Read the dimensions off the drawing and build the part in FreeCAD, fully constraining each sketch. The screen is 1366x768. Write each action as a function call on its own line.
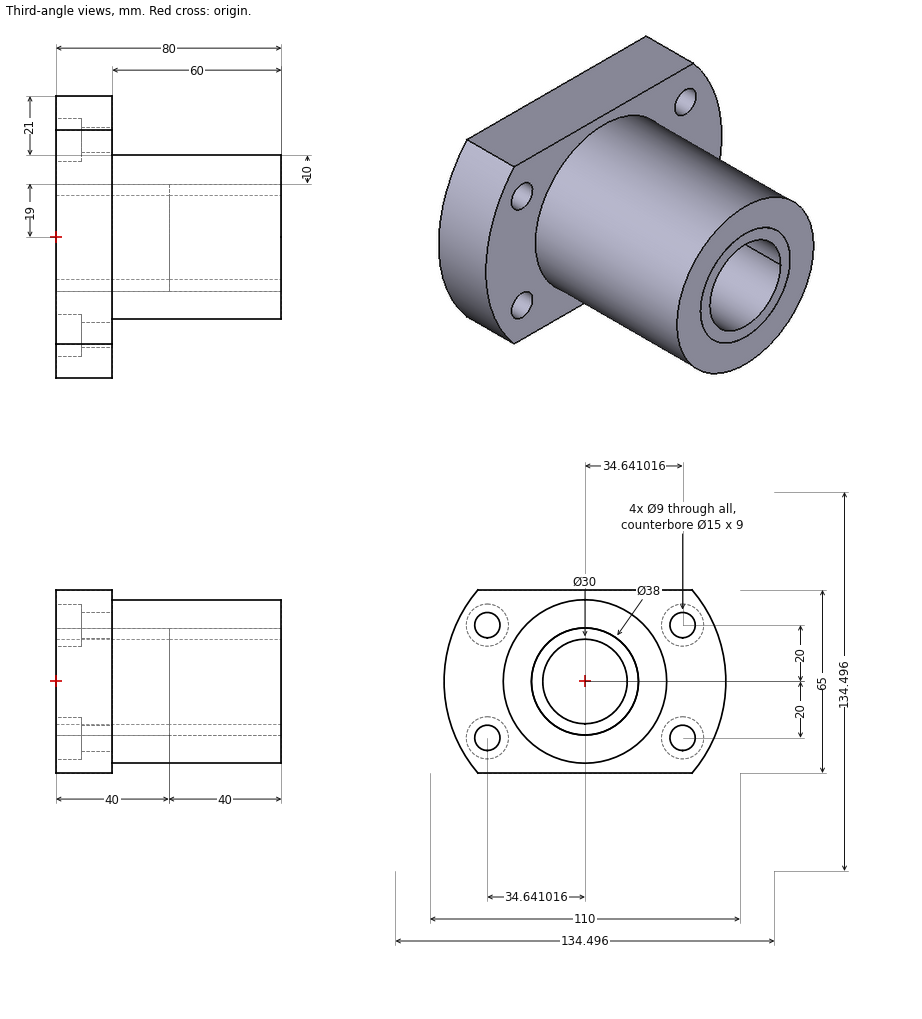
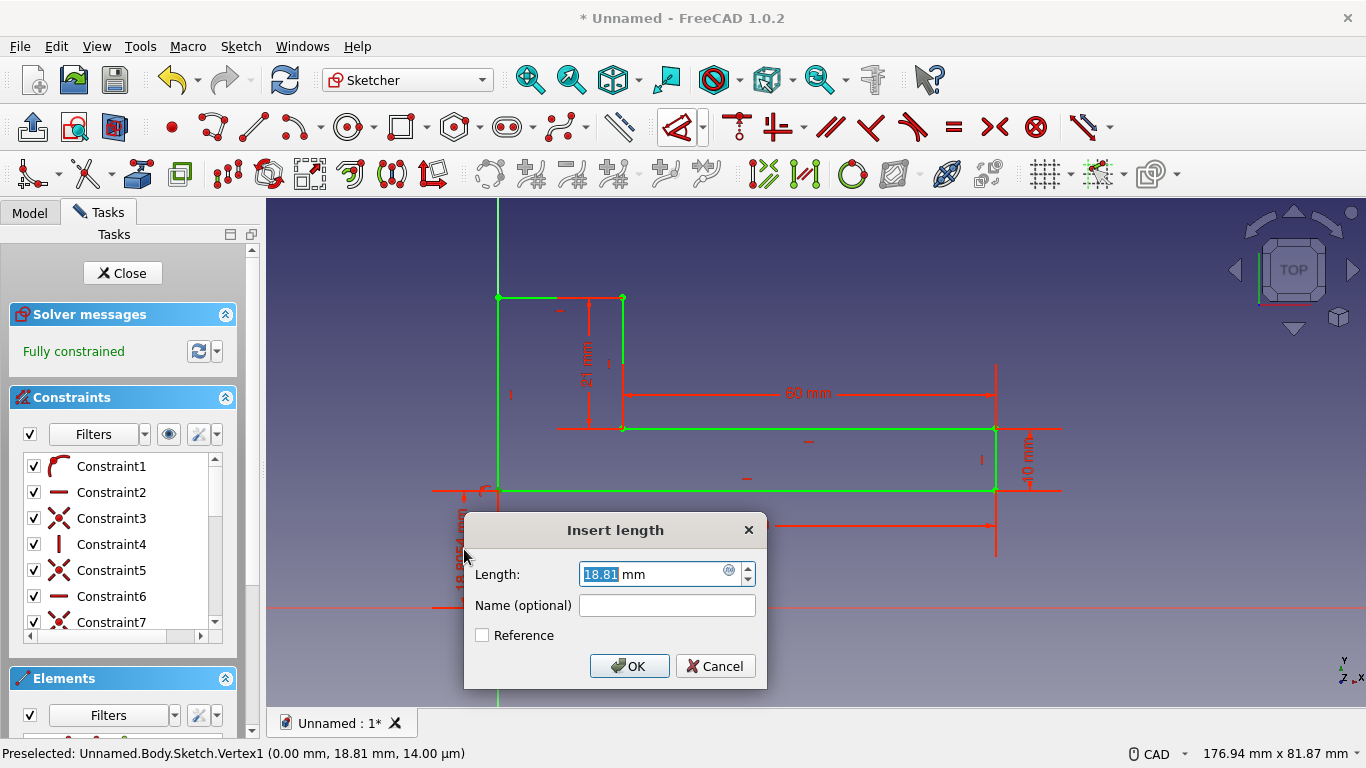
text(19)
key(Return)
key(Escape)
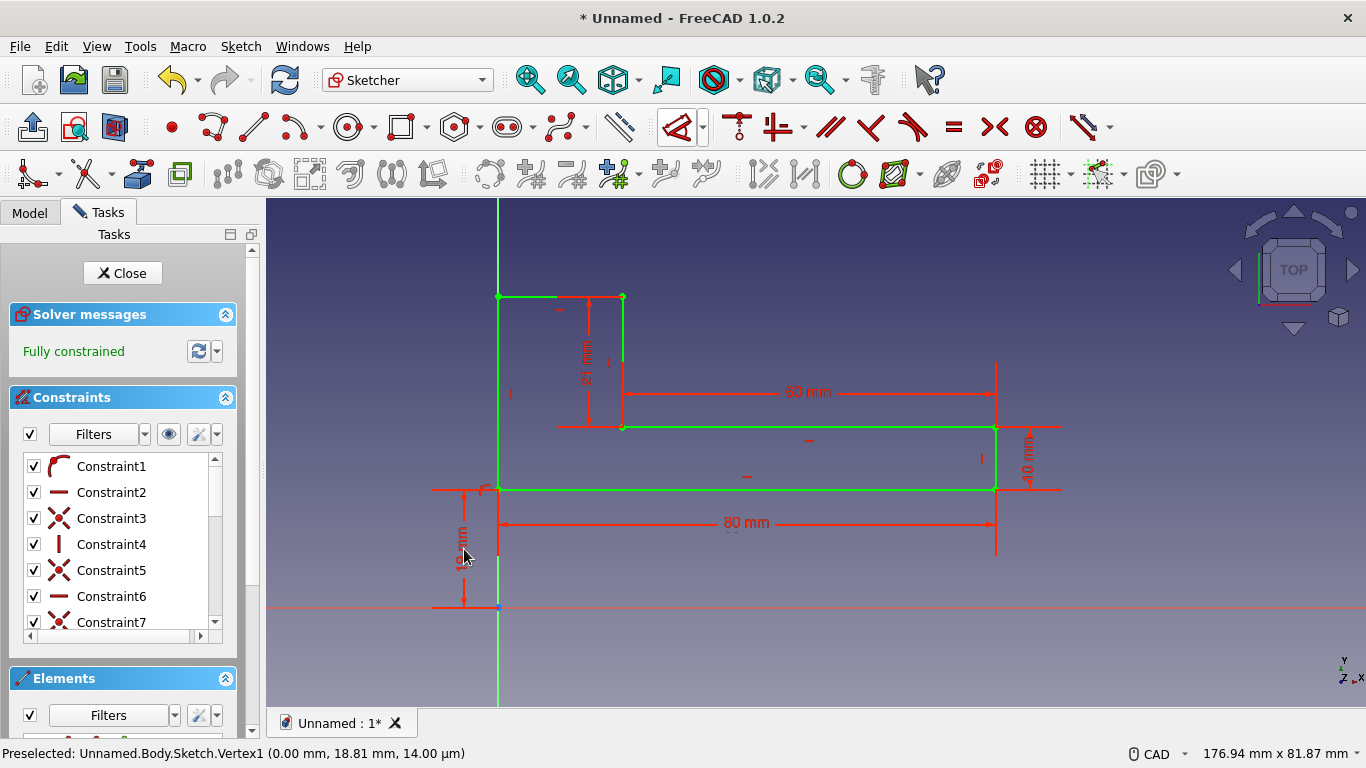
click(123, 273)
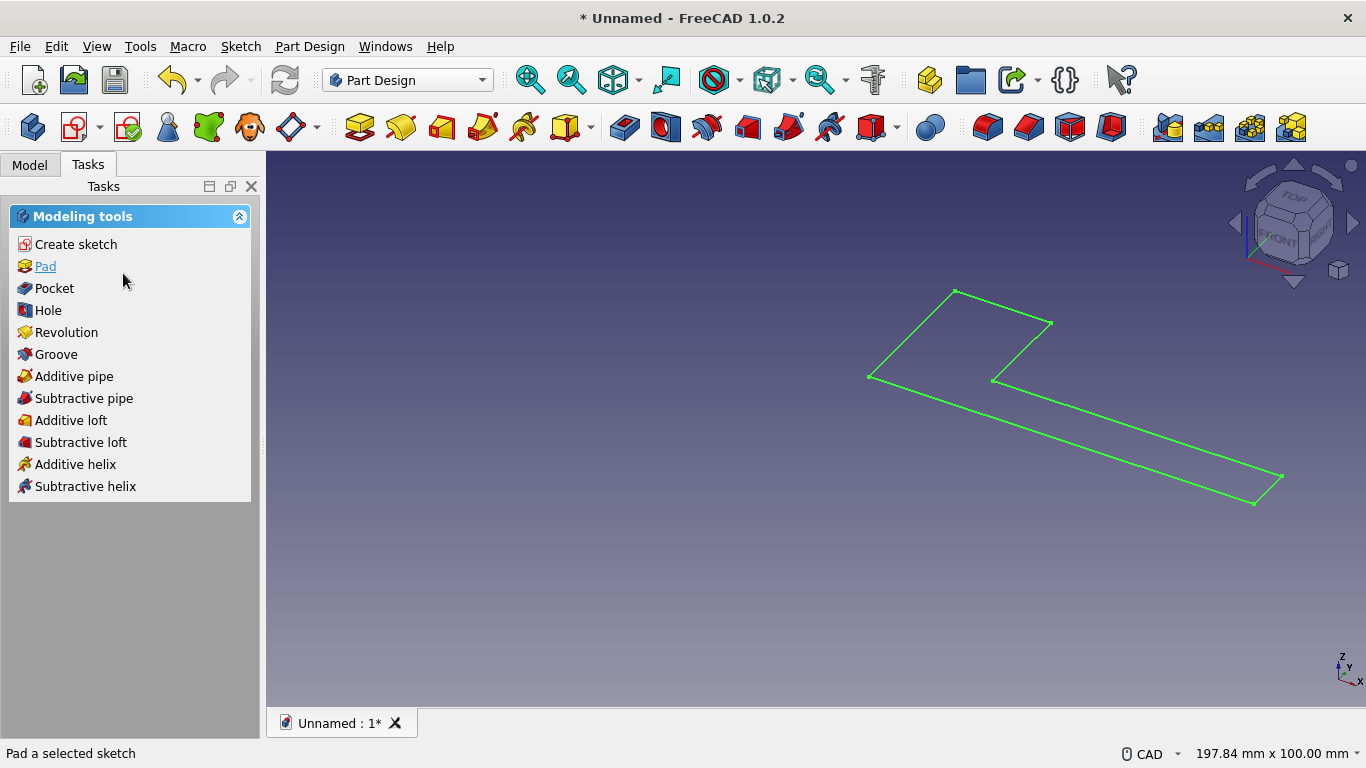
click(401, 128)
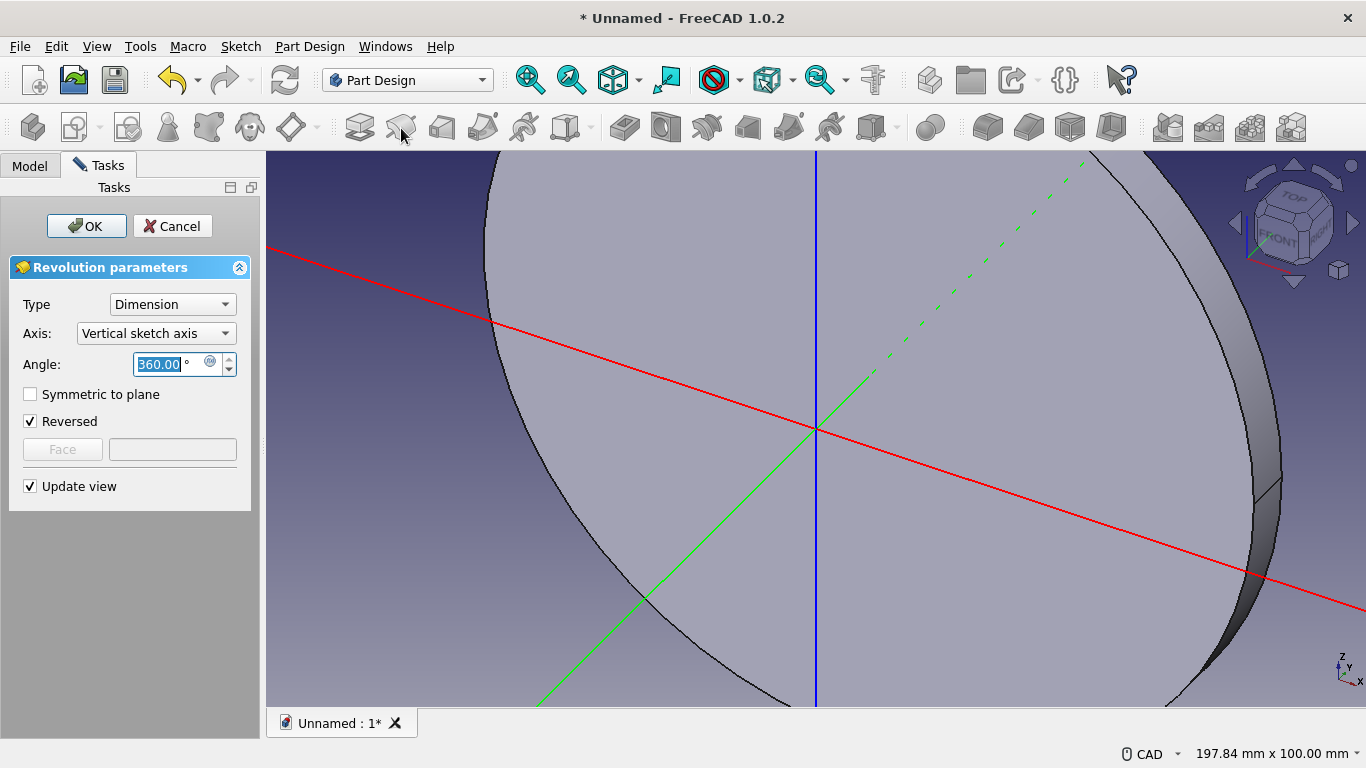
click(157, 334)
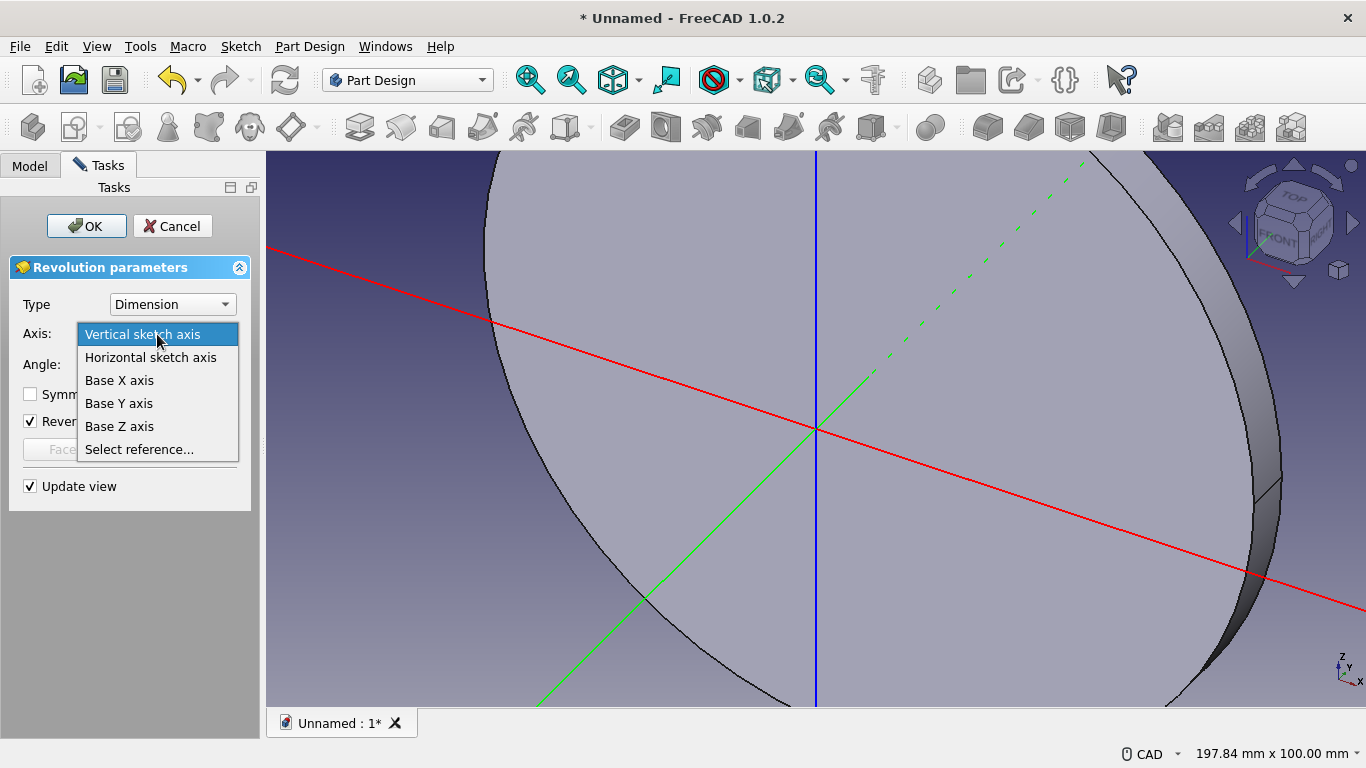
click(156, 358)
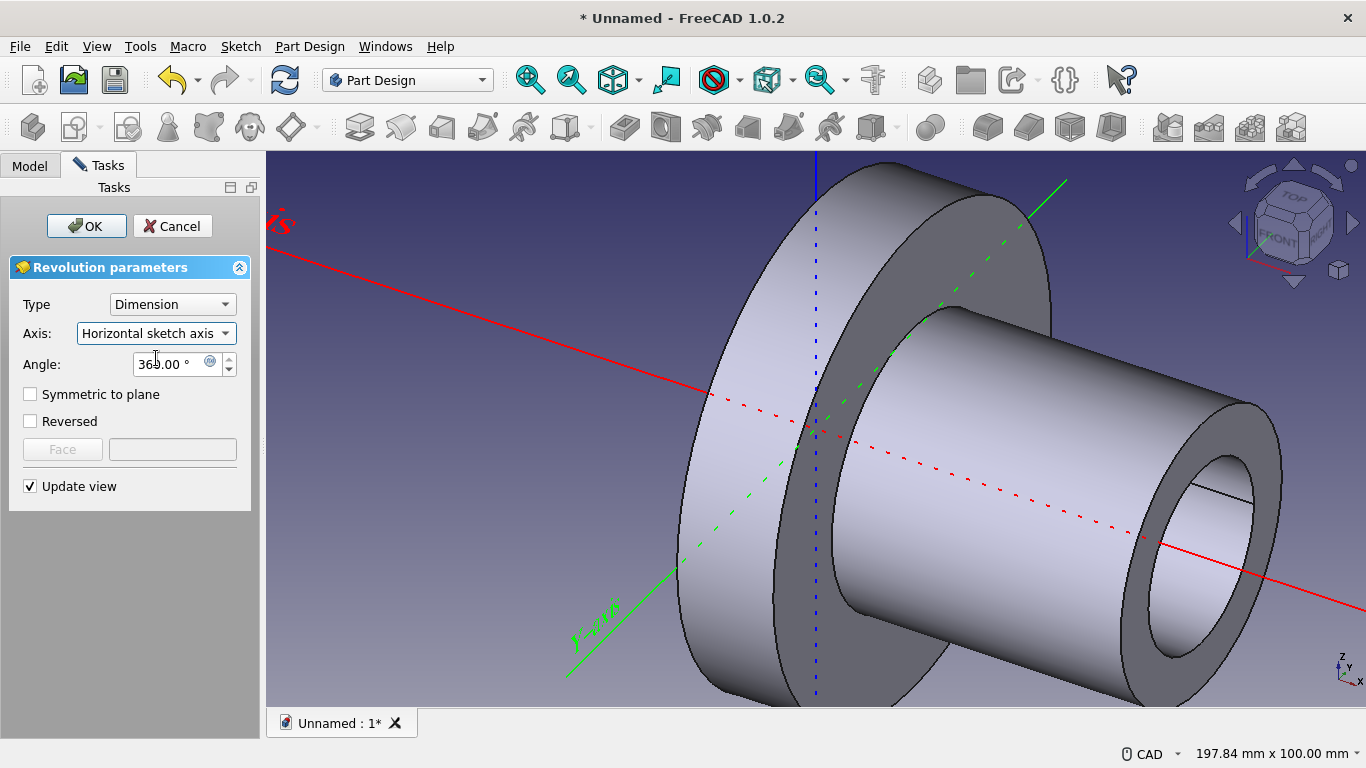
click(87, 226)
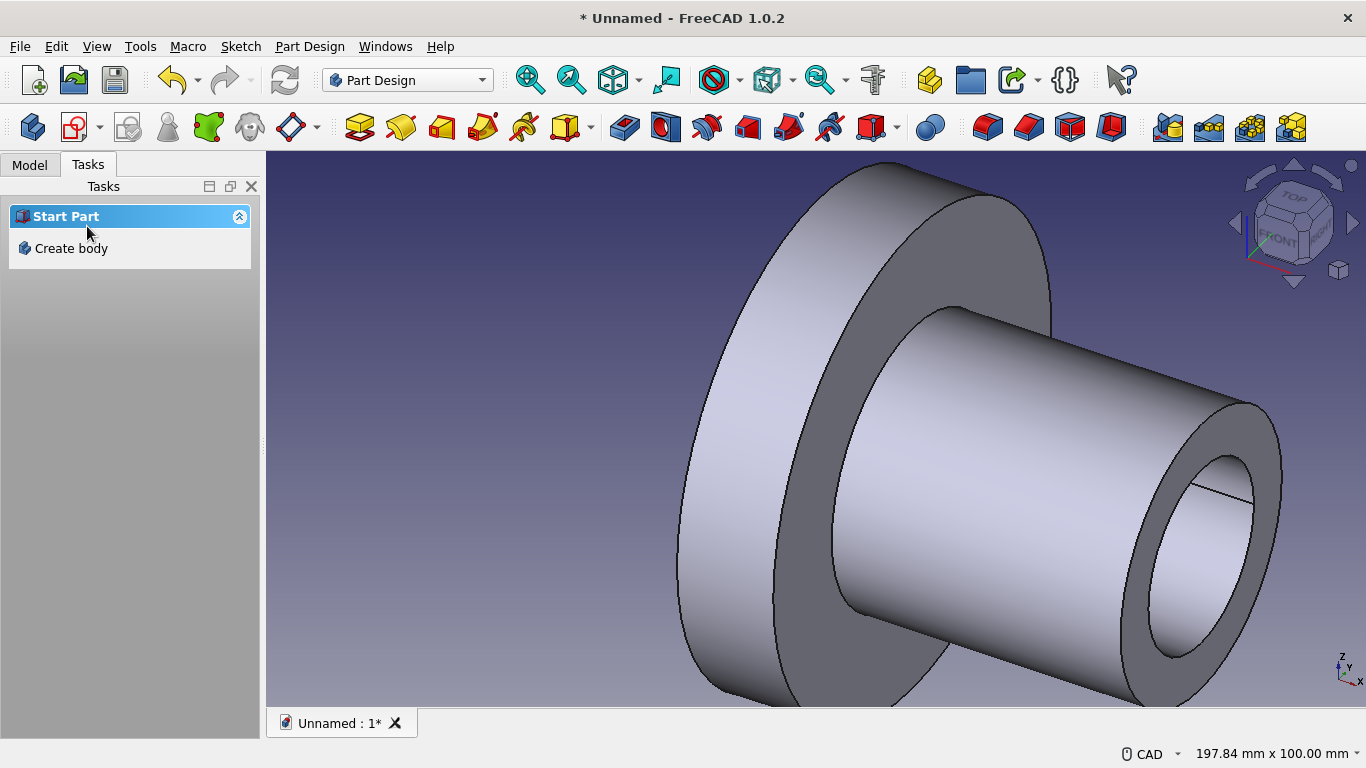
click(531, 80)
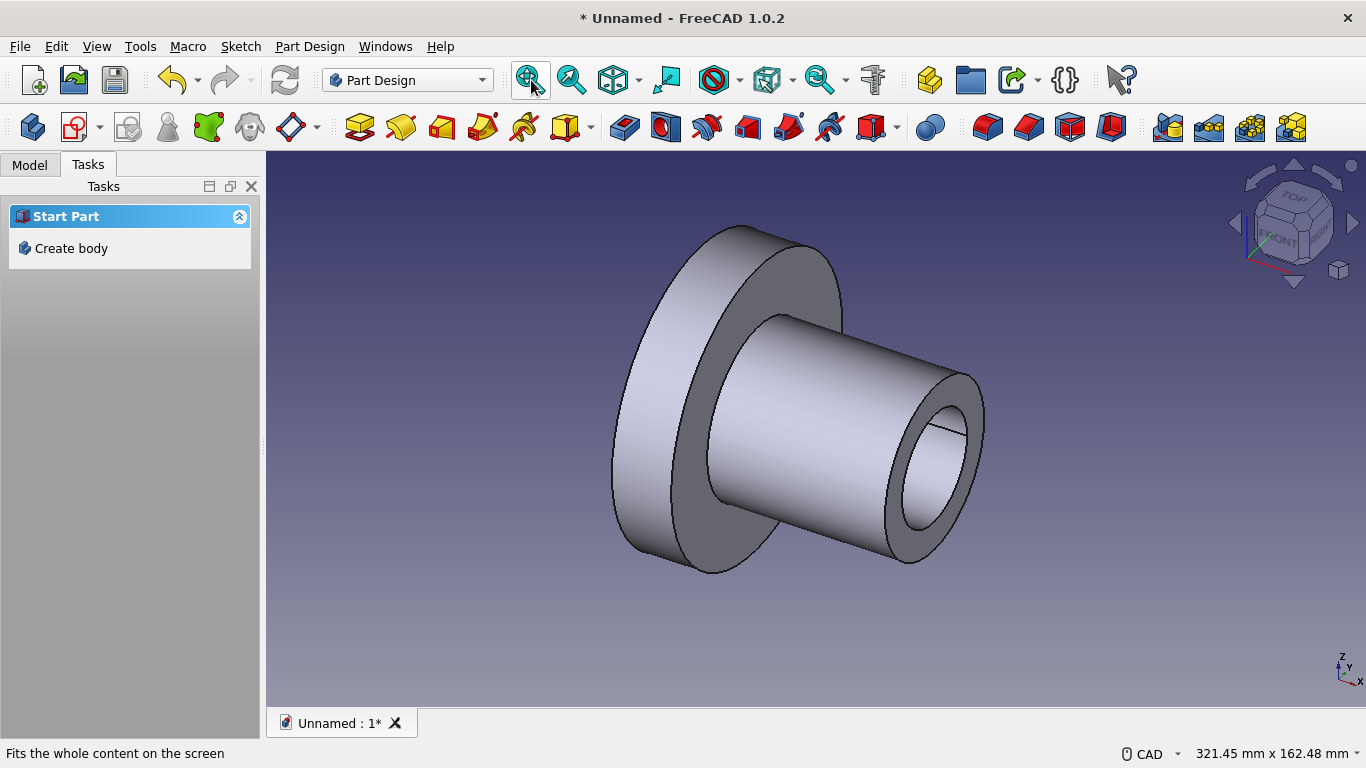
click(74, 128)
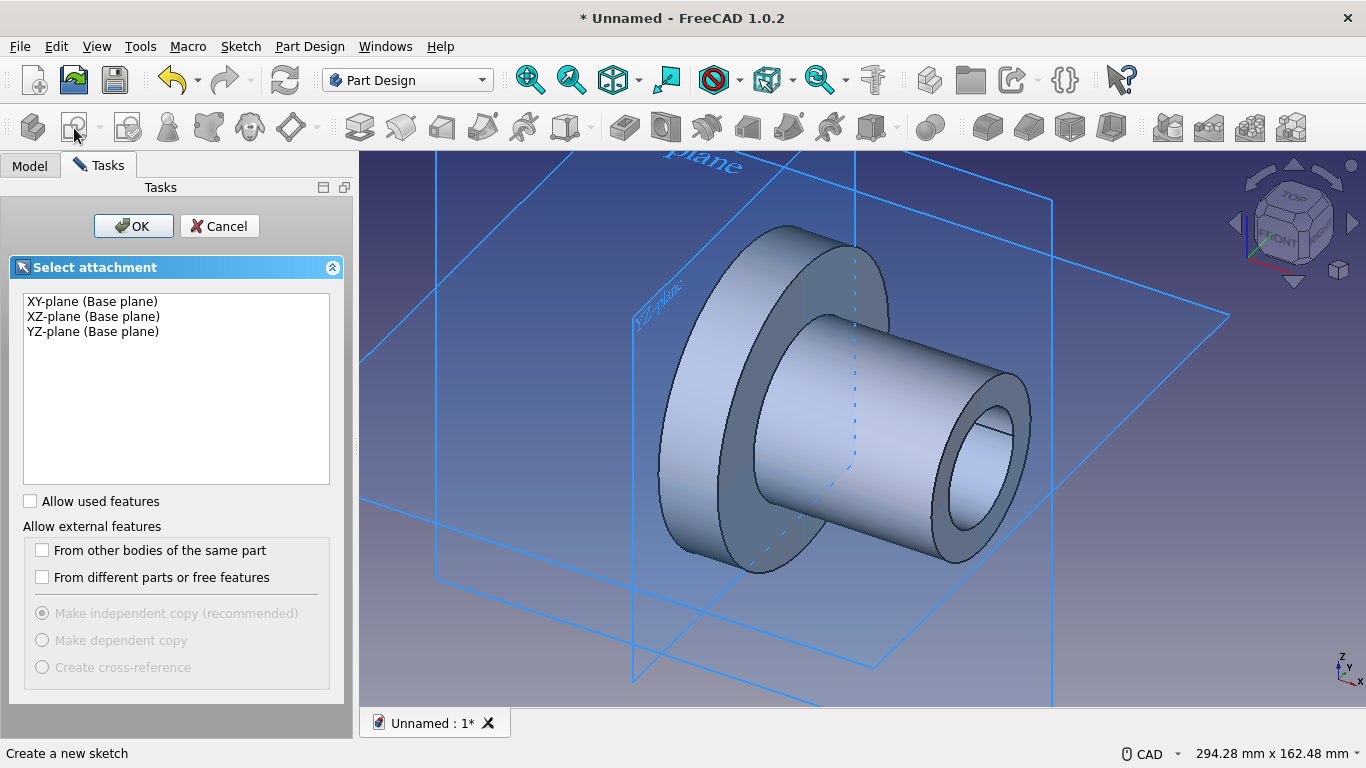
click(84, 332)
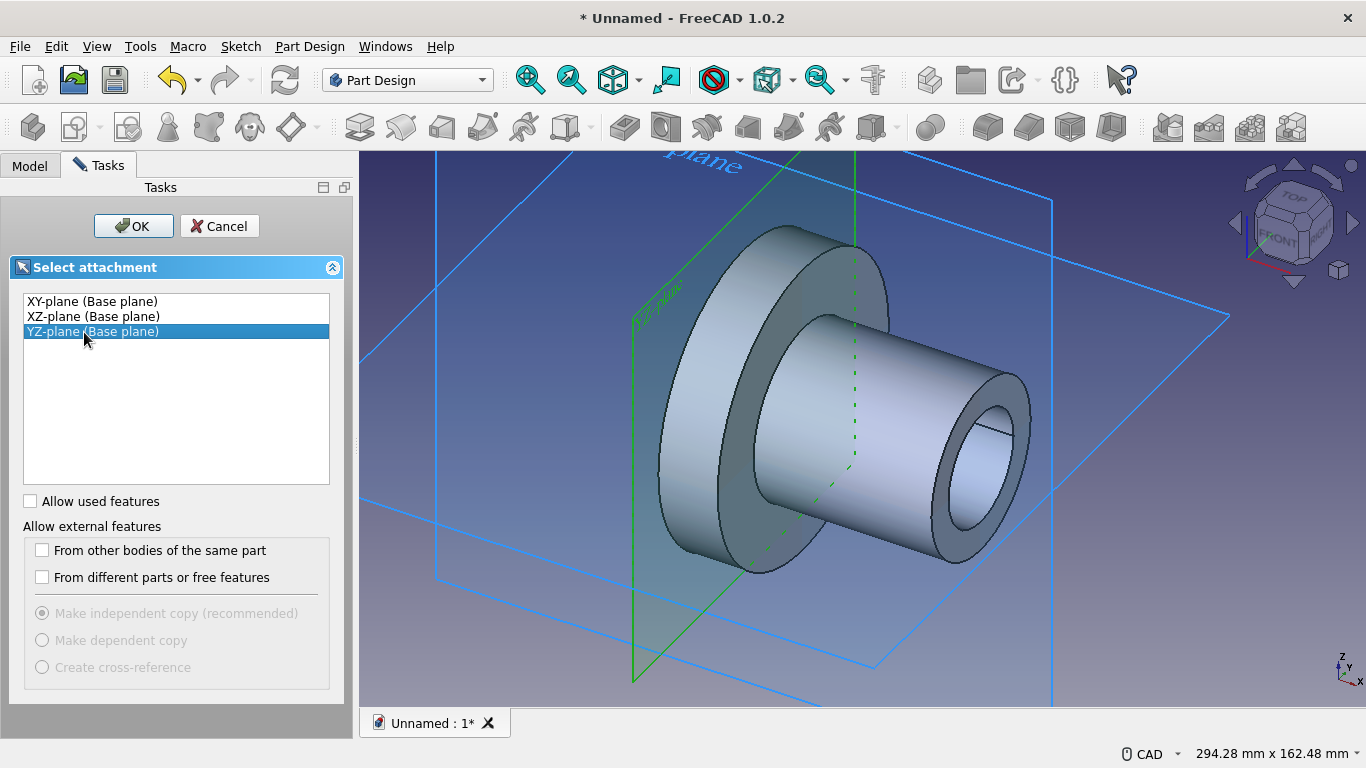
click(134, 226)